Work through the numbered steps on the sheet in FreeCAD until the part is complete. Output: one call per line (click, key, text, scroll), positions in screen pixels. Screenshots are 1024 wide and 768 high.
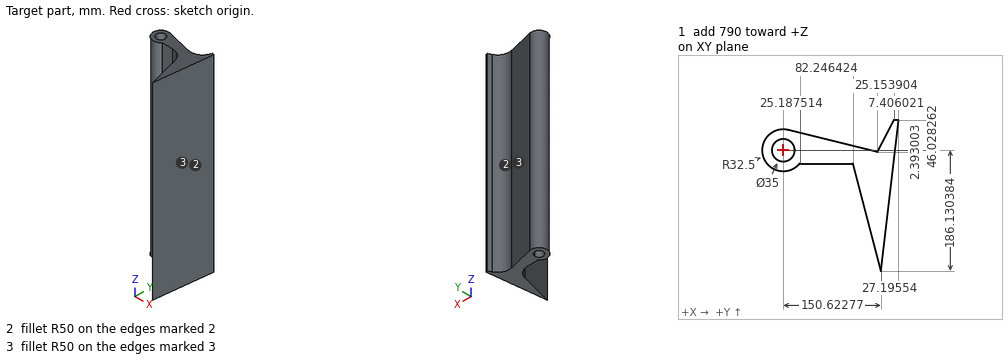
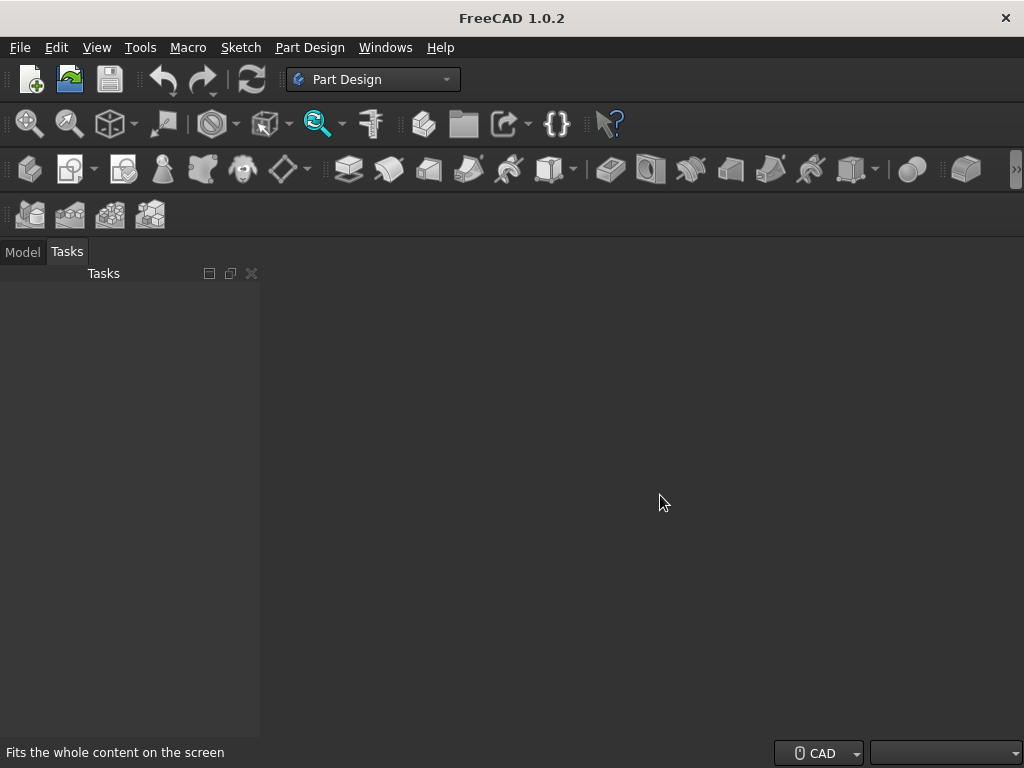
key(ctrl+n)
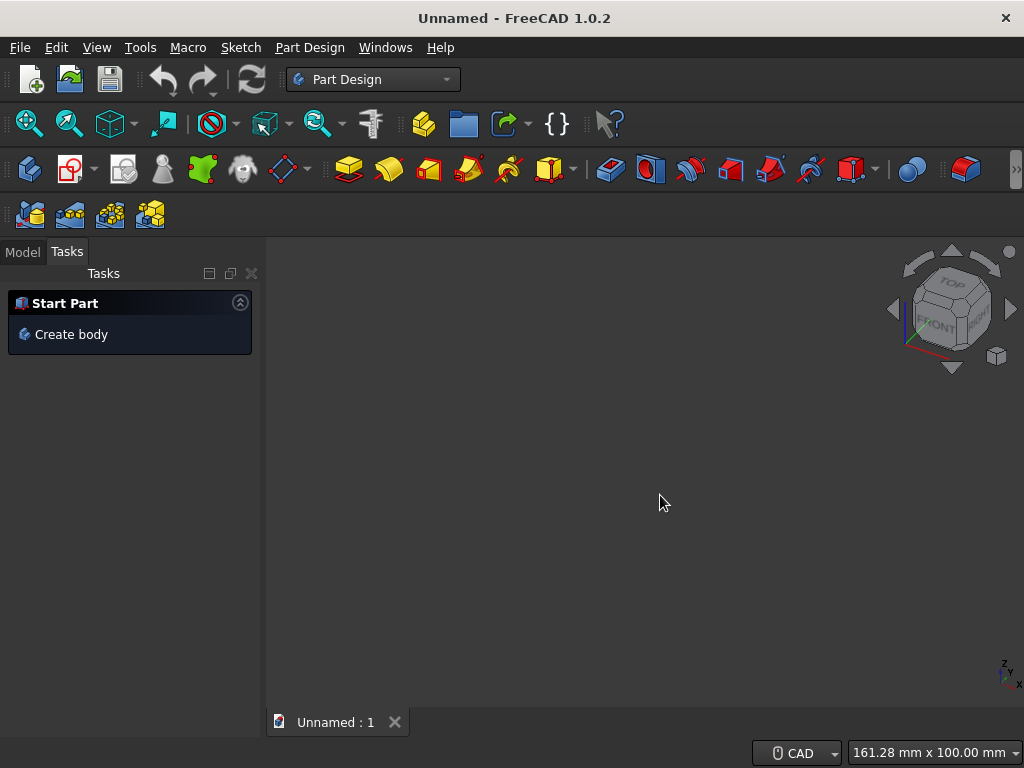
click(70, 170)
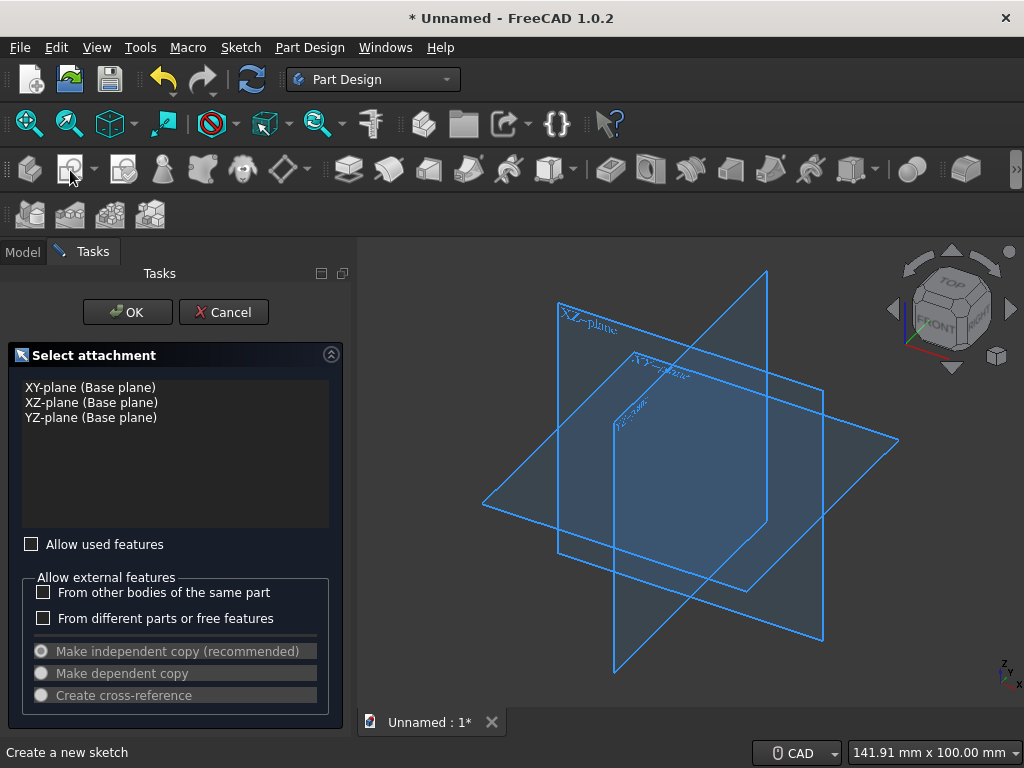
click(82, 388)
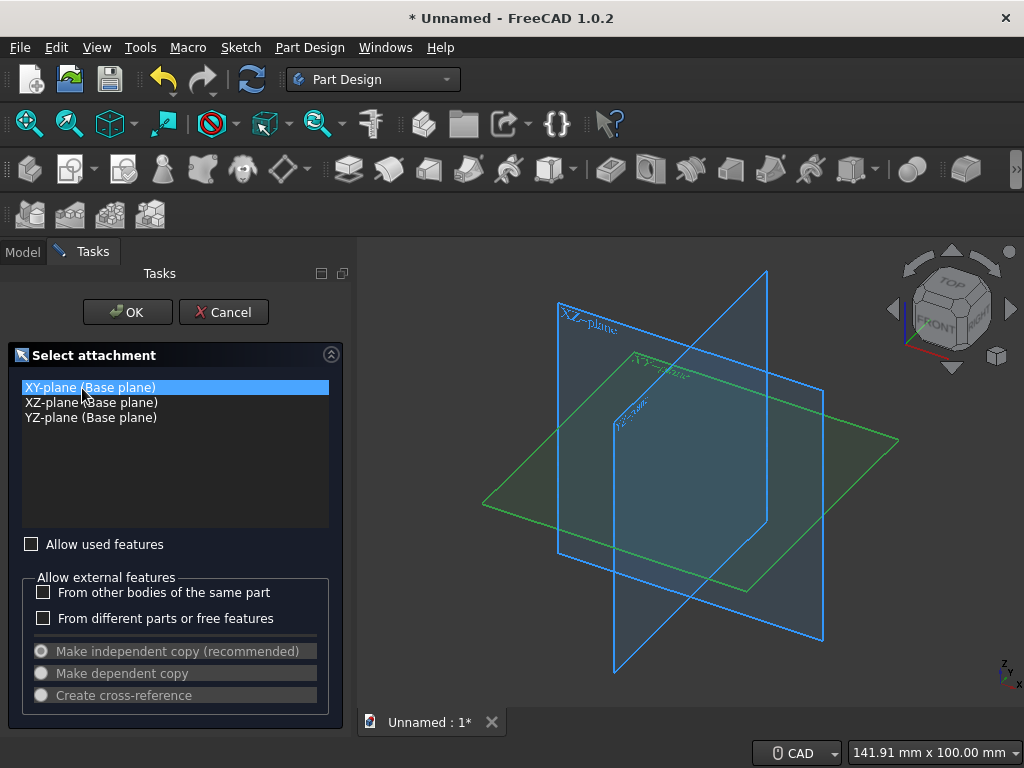
click(128, 312)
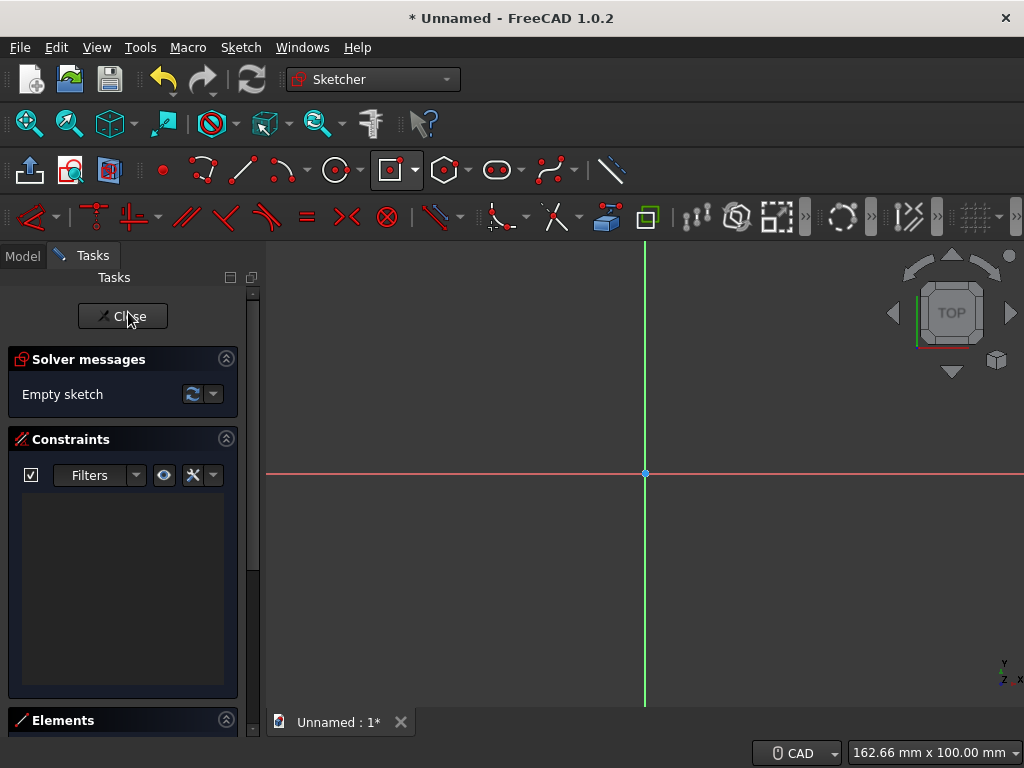
scroll(442, 367, down, 7)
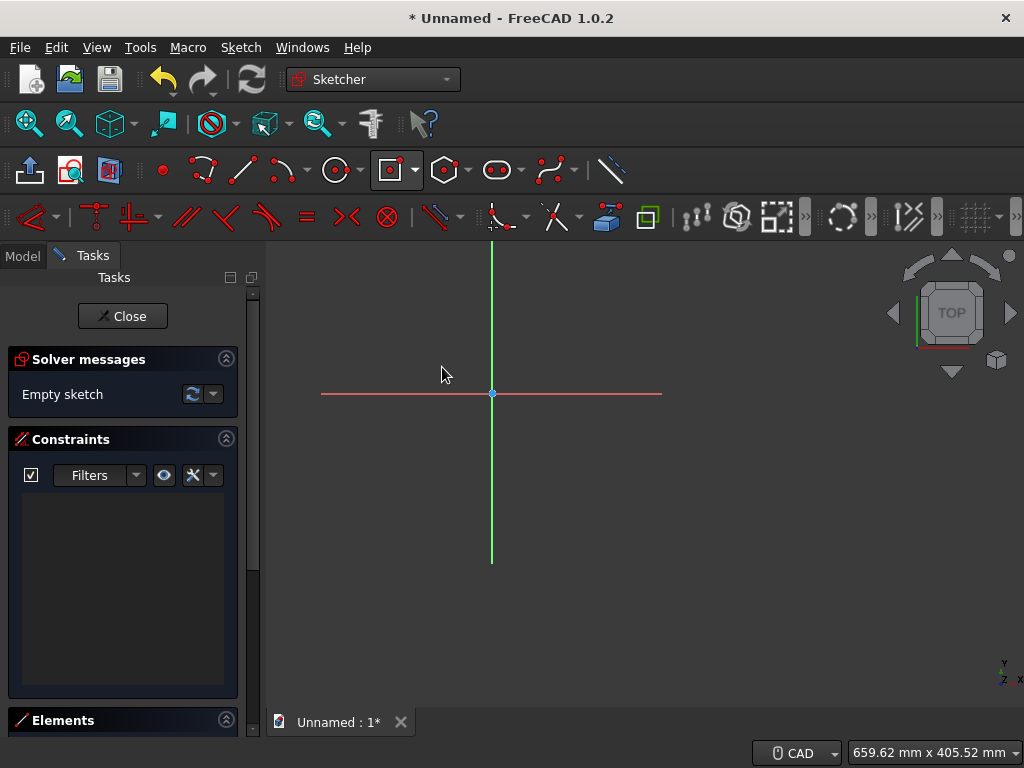
key(g)
key(m)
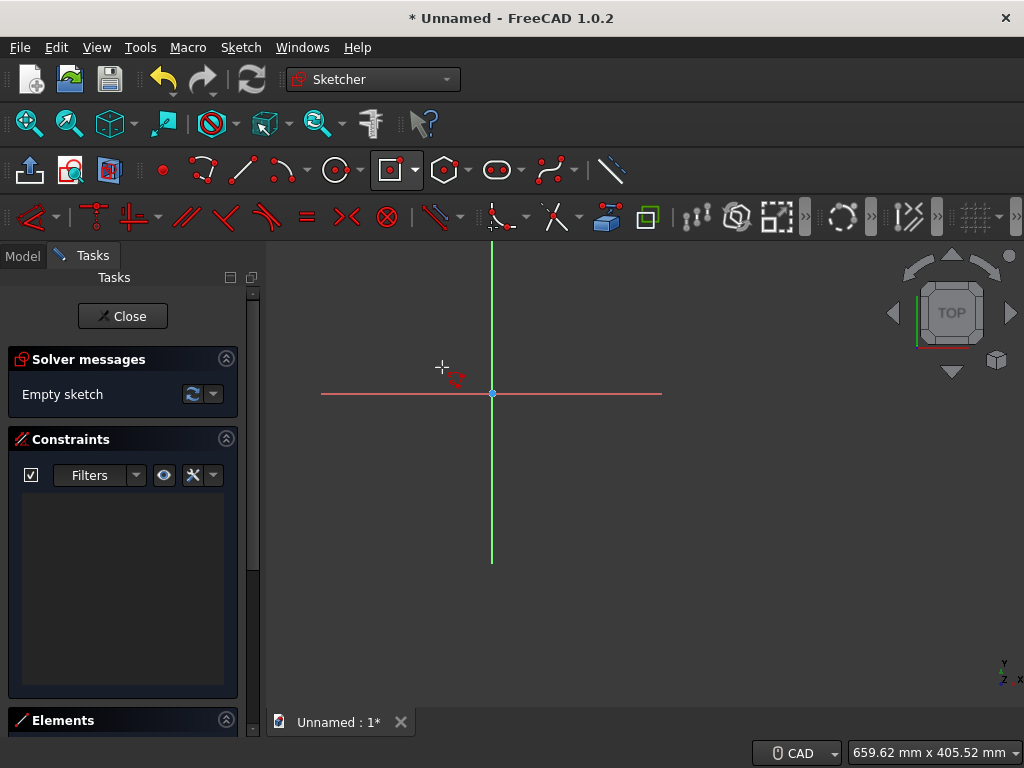
click(521, 417)
click(616, 417)
click(665, 607)
click(697, 341)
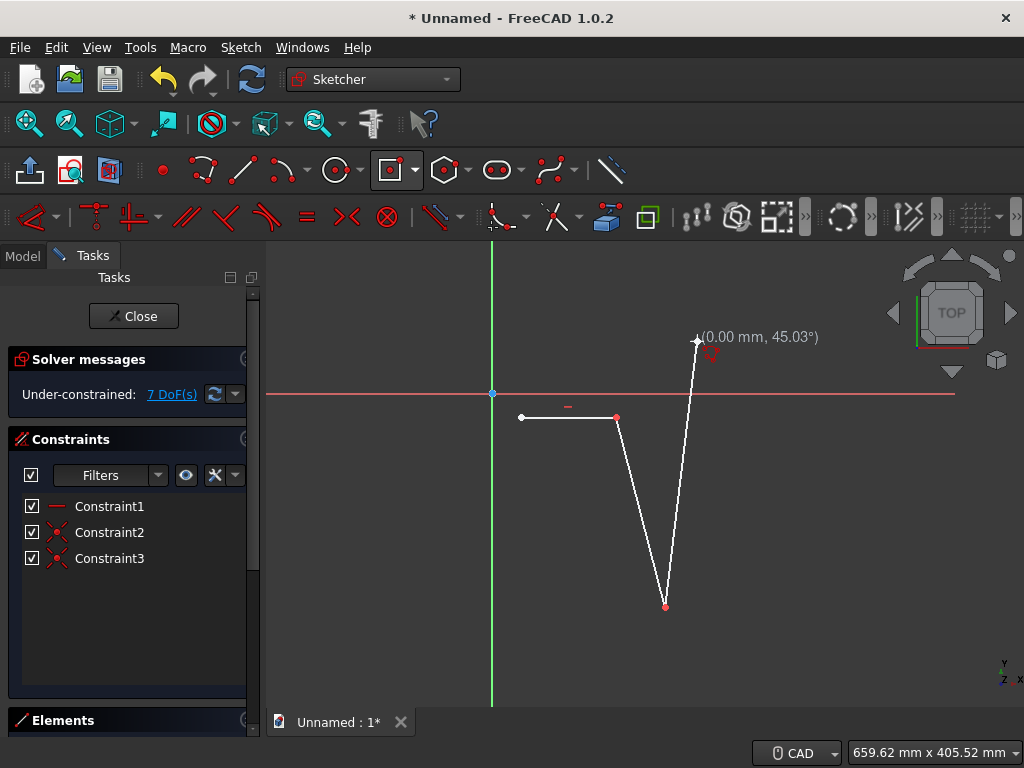
scroll(688, 341, up, 4)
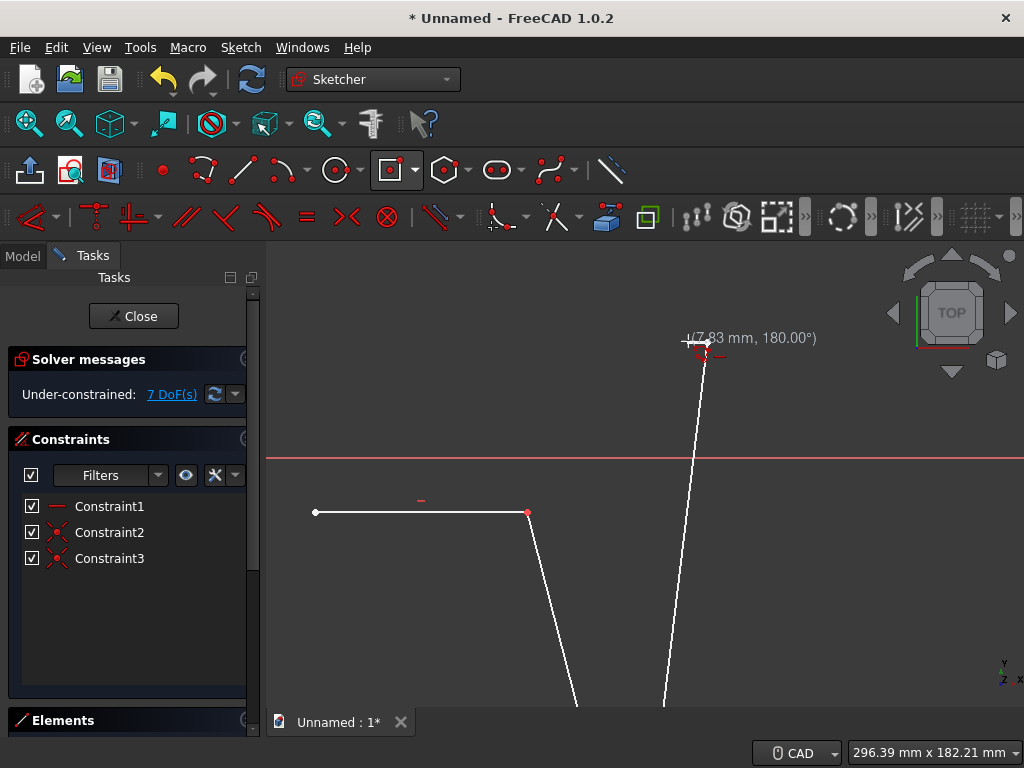
click(687, 341)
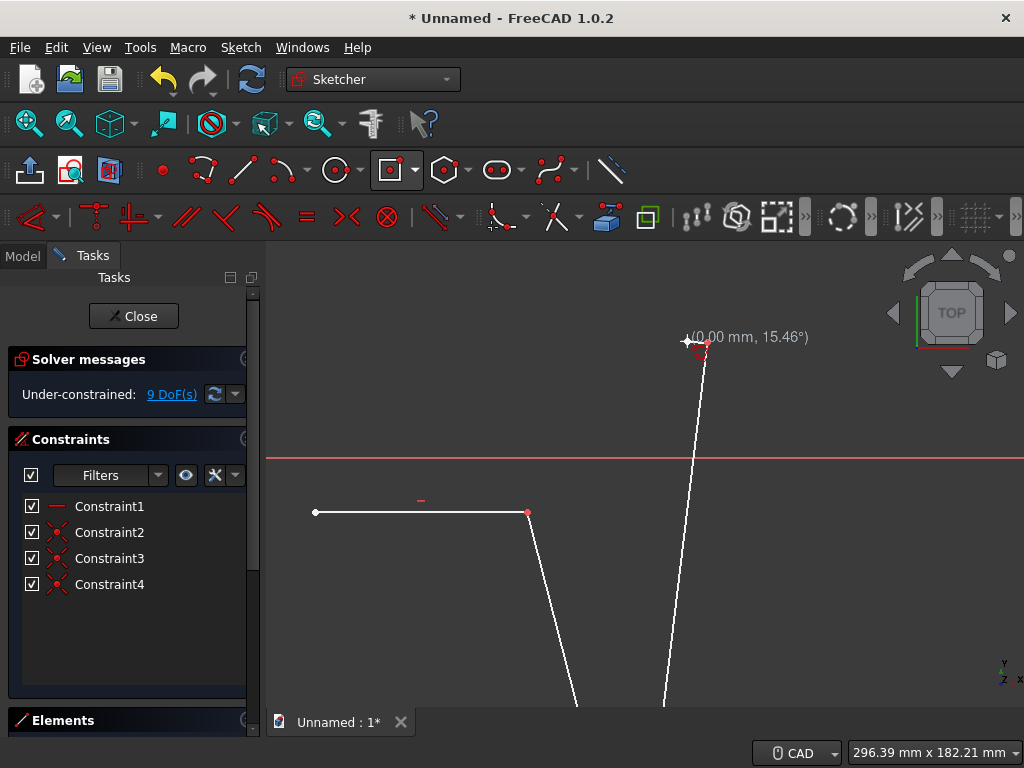
scroll(623, 464, up, 5)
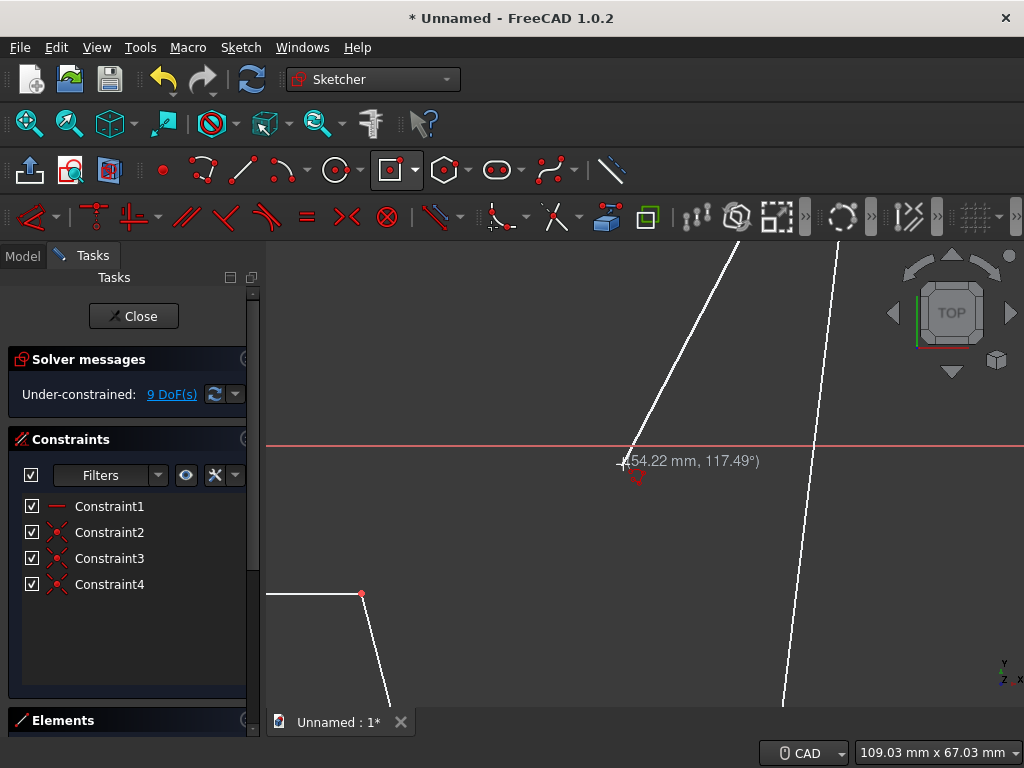
click(623, 463)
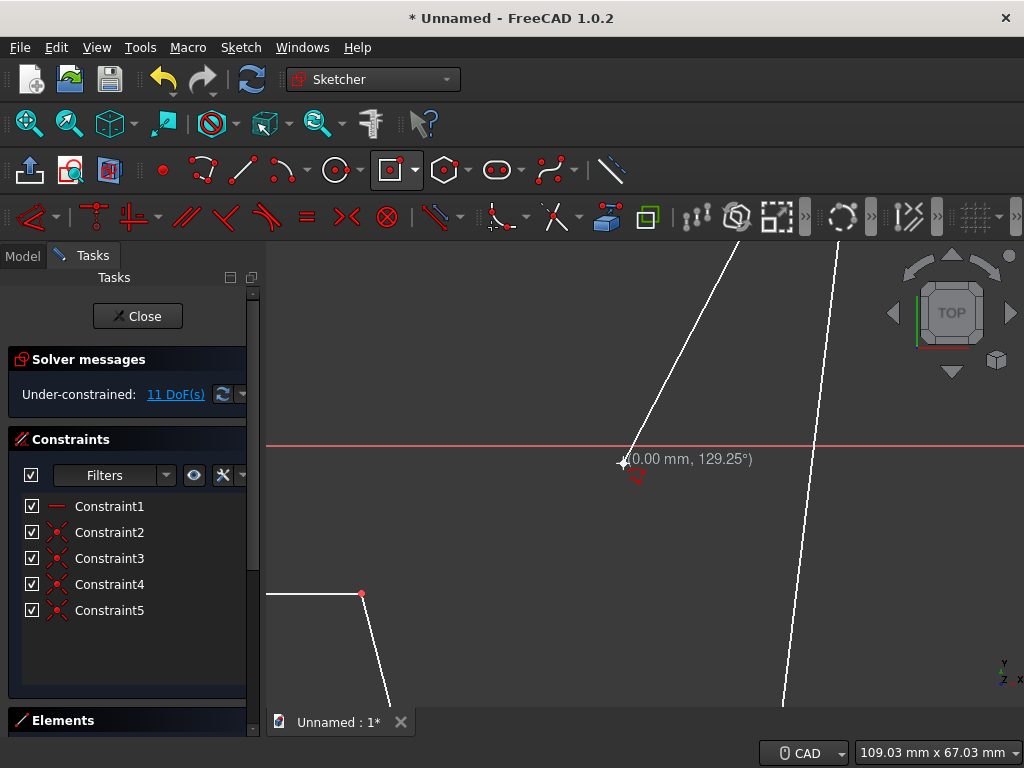
scroll(666, 383, down, 9)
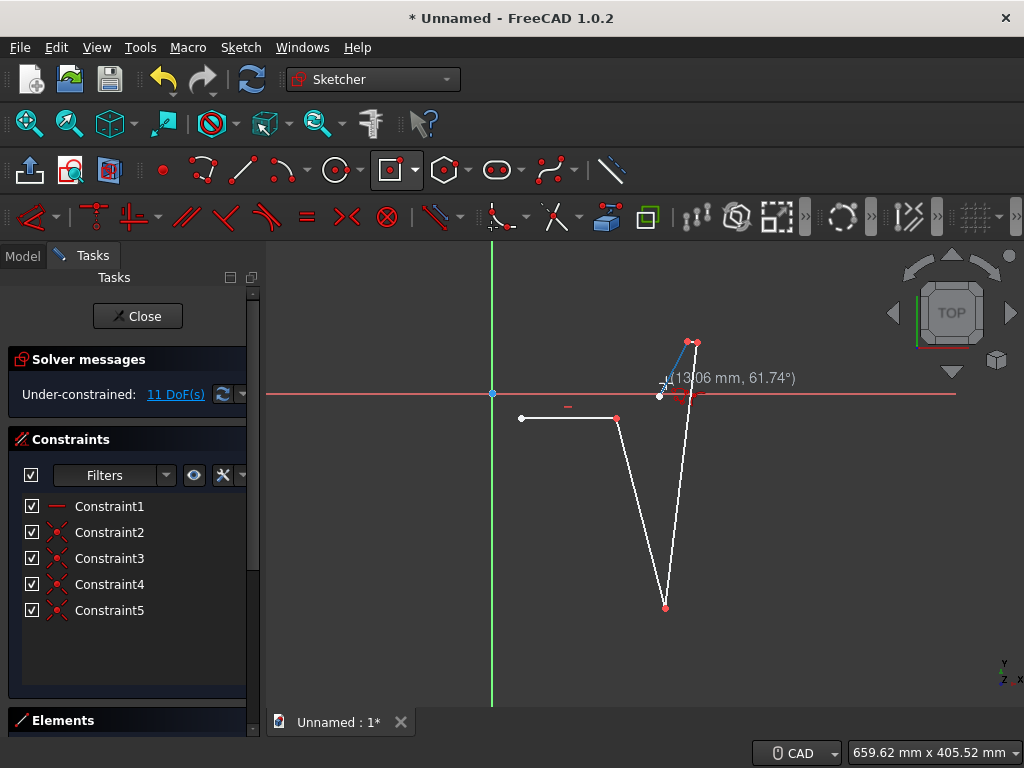
scroll(501, 357, up, 3)